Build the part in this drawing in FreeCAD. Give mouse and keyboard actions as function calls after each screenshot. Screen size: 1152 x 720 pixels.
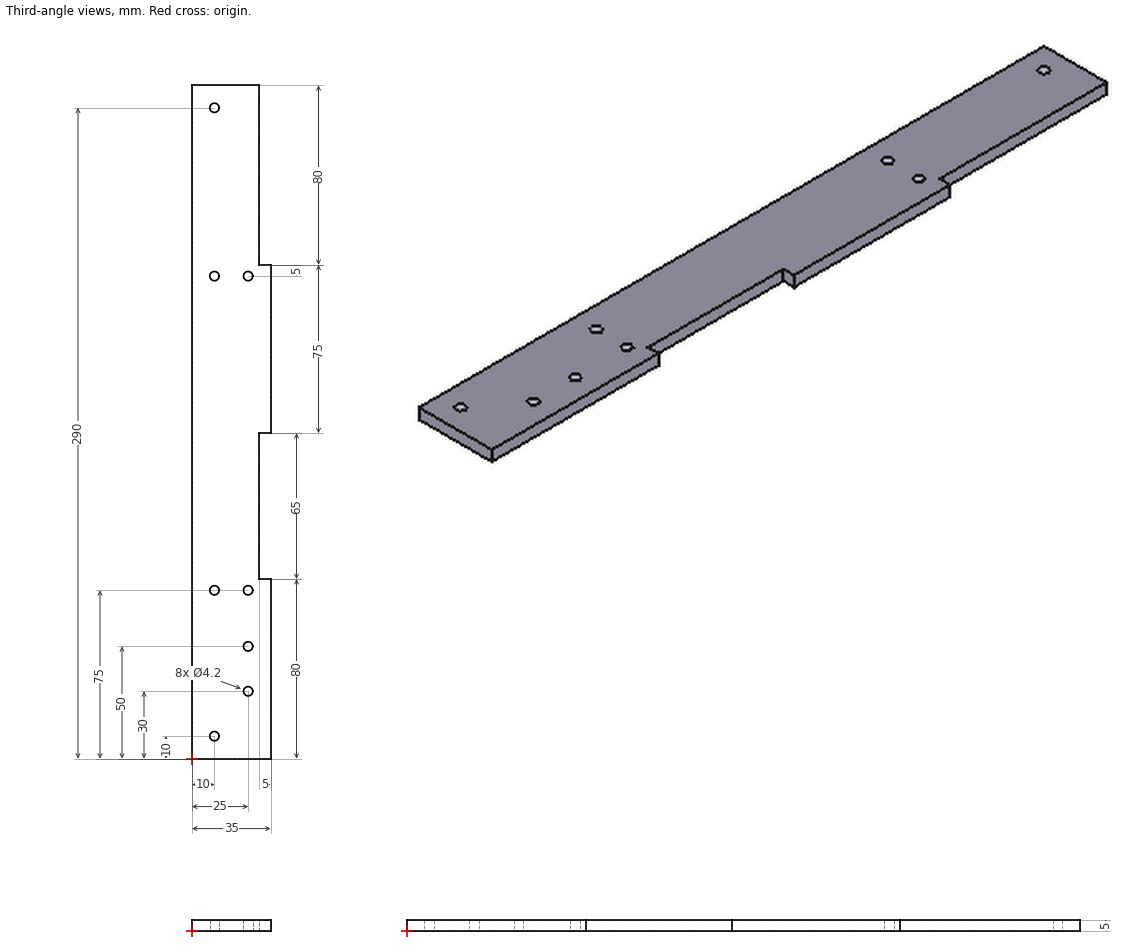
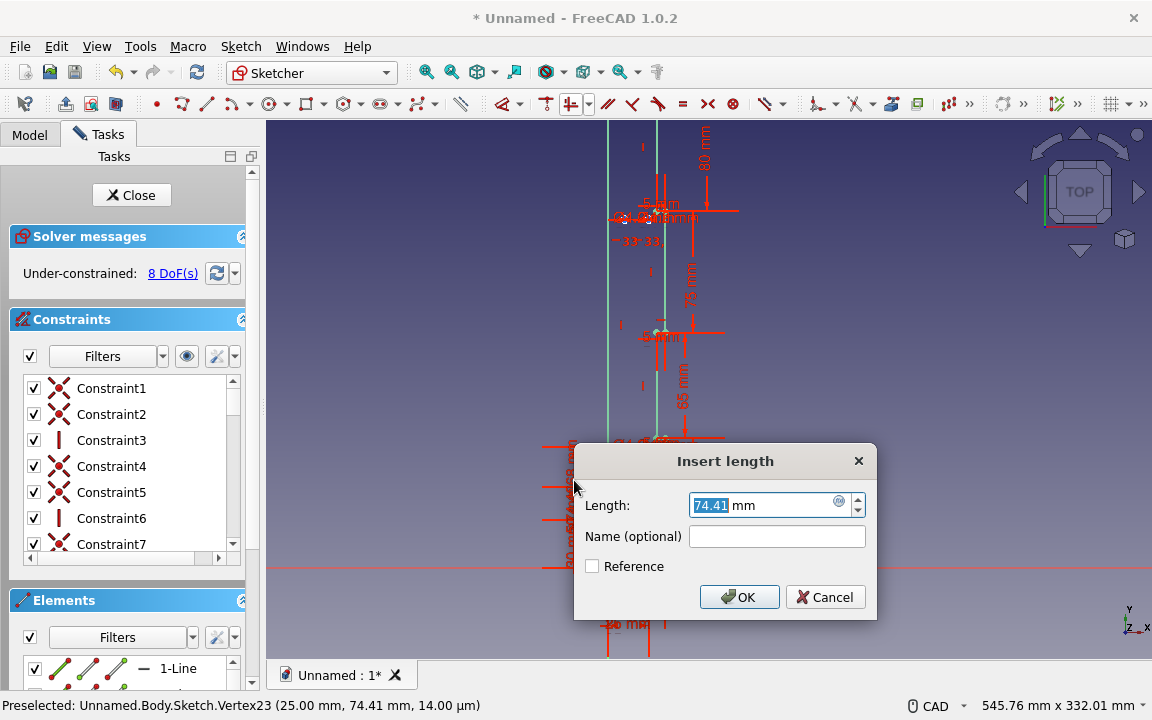
text(75)
key(Return)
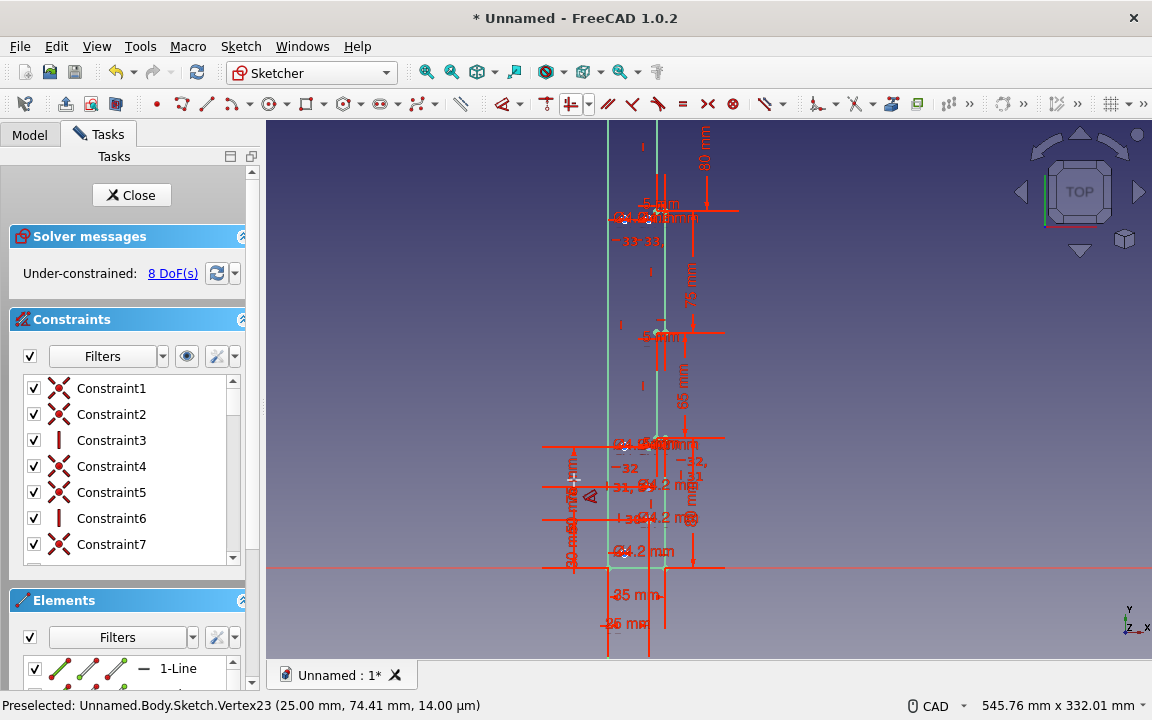
scroll(625, 553, up, 5)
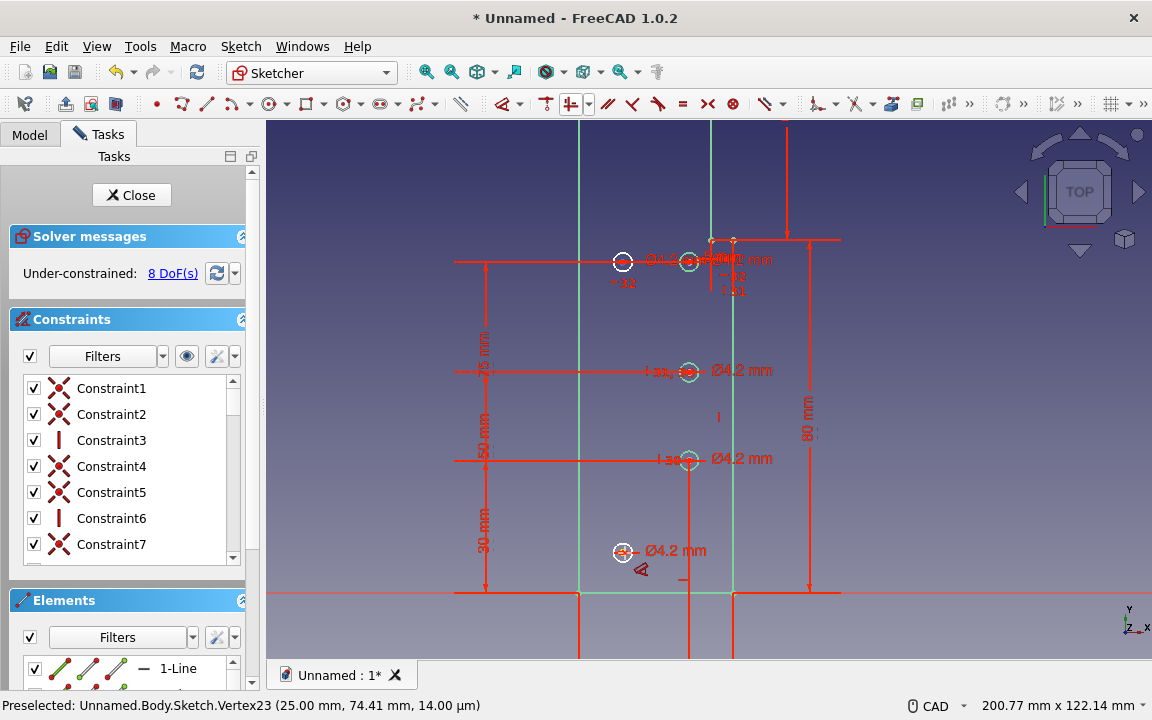
click(623, 553)
click(601, 627)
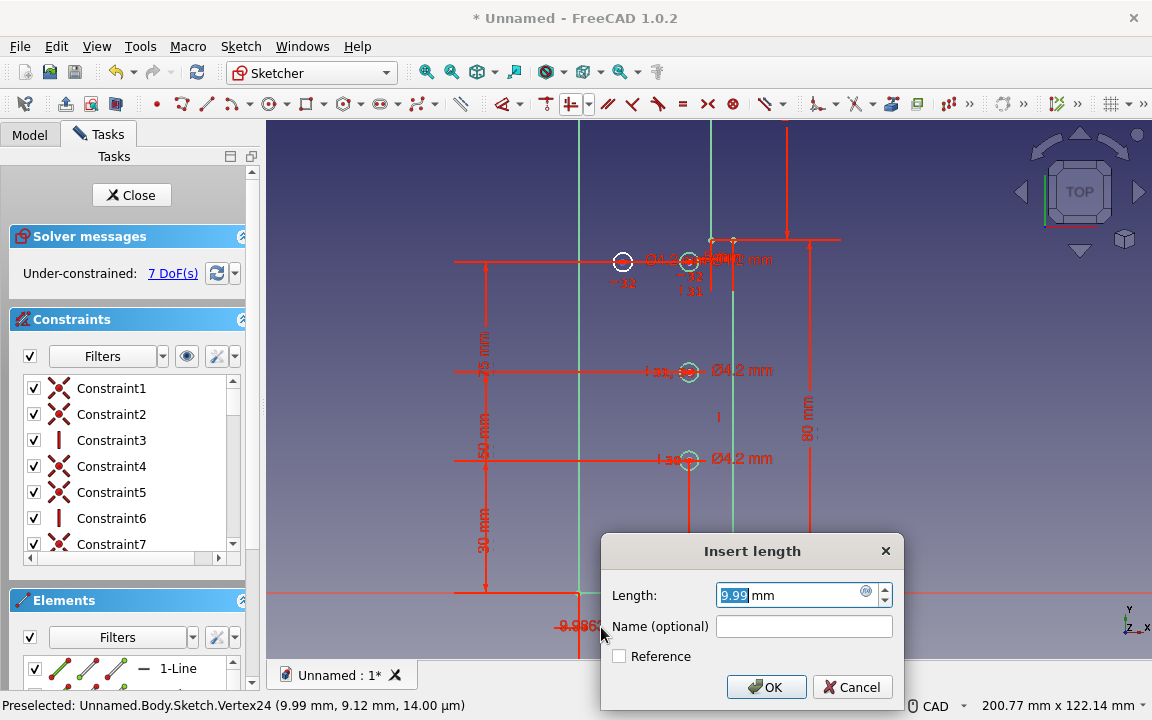
text(10)
key(Return)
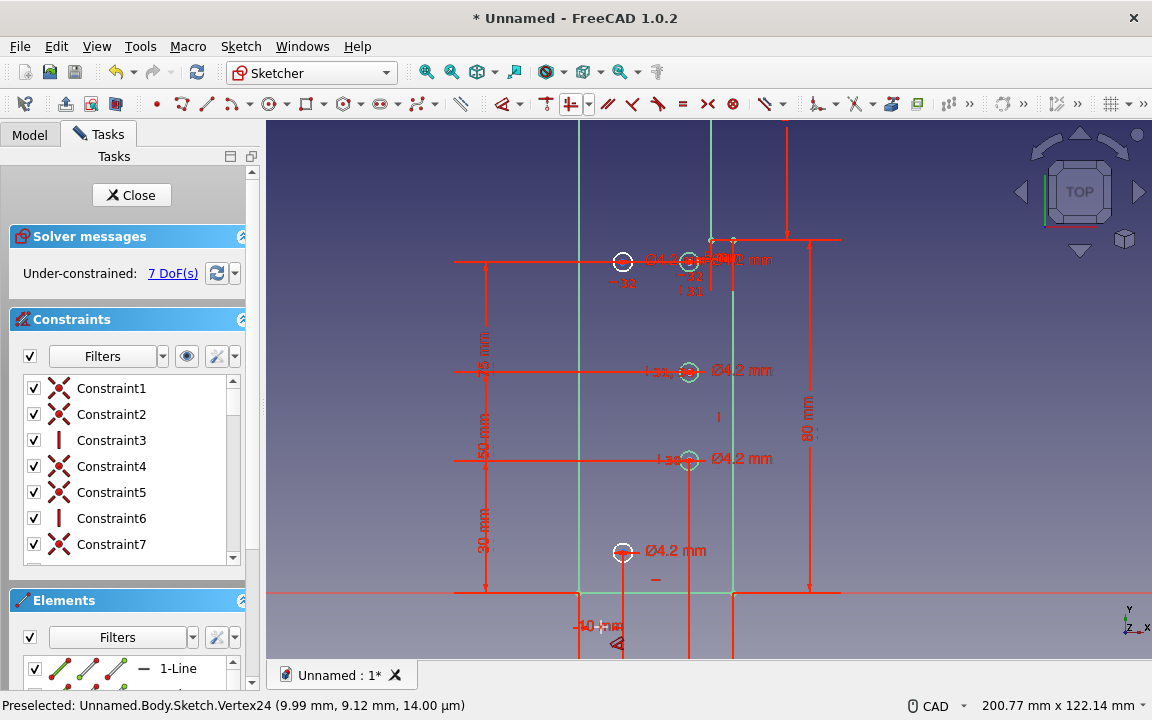
click(623, 553)
click(545, 573)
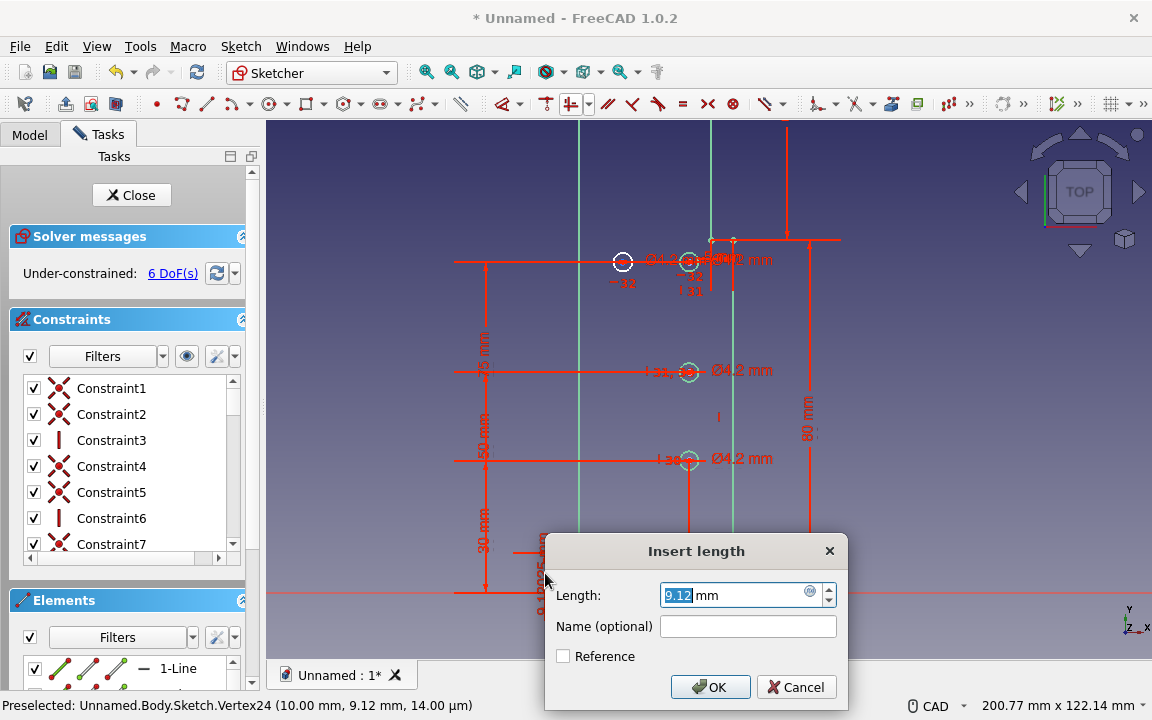
text(10)
key(Return)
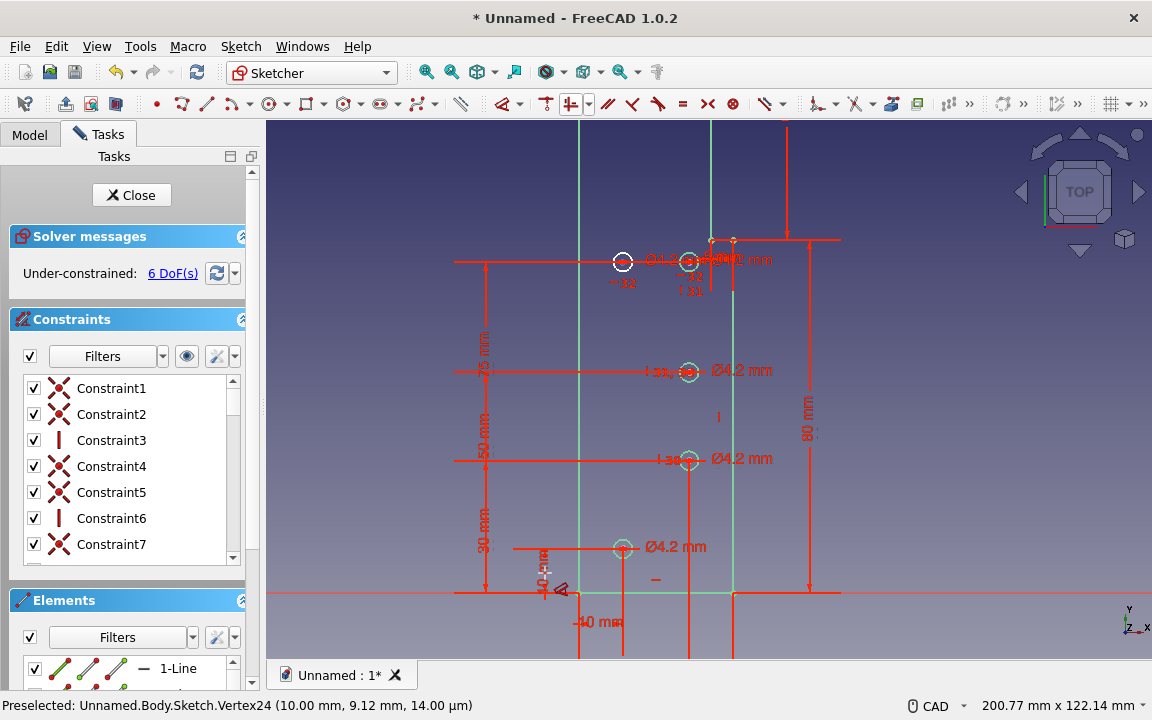
click(623, 262)
click(601, 228)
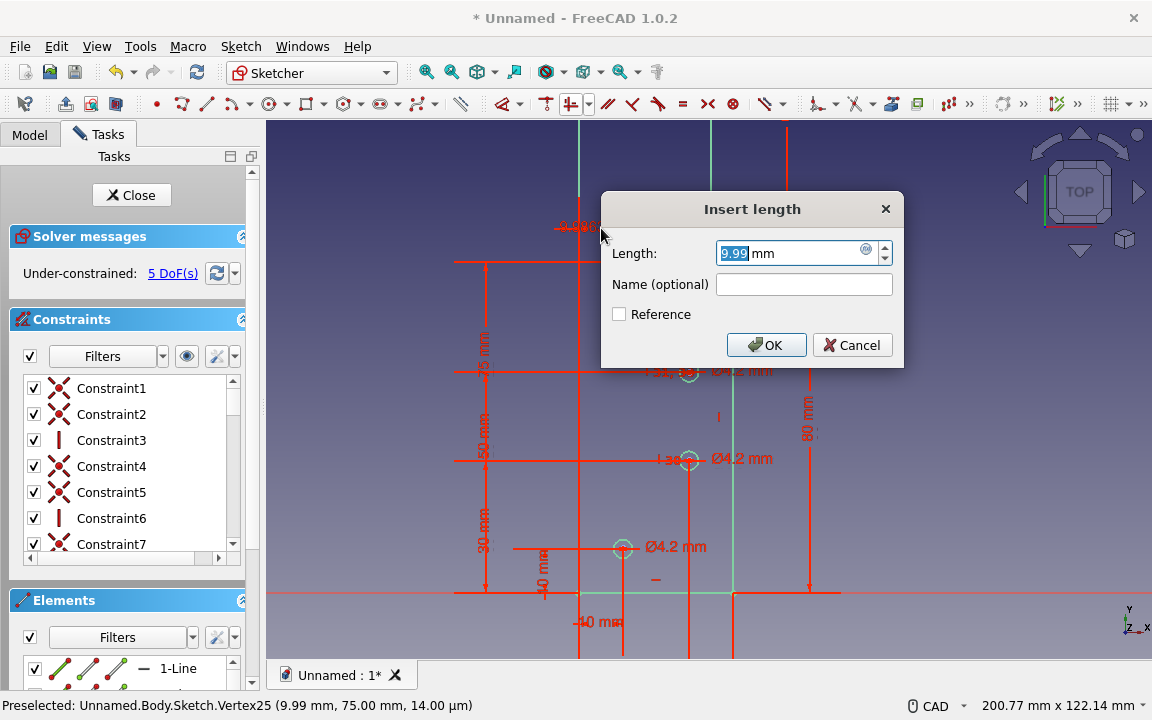
text(10)
key(Return)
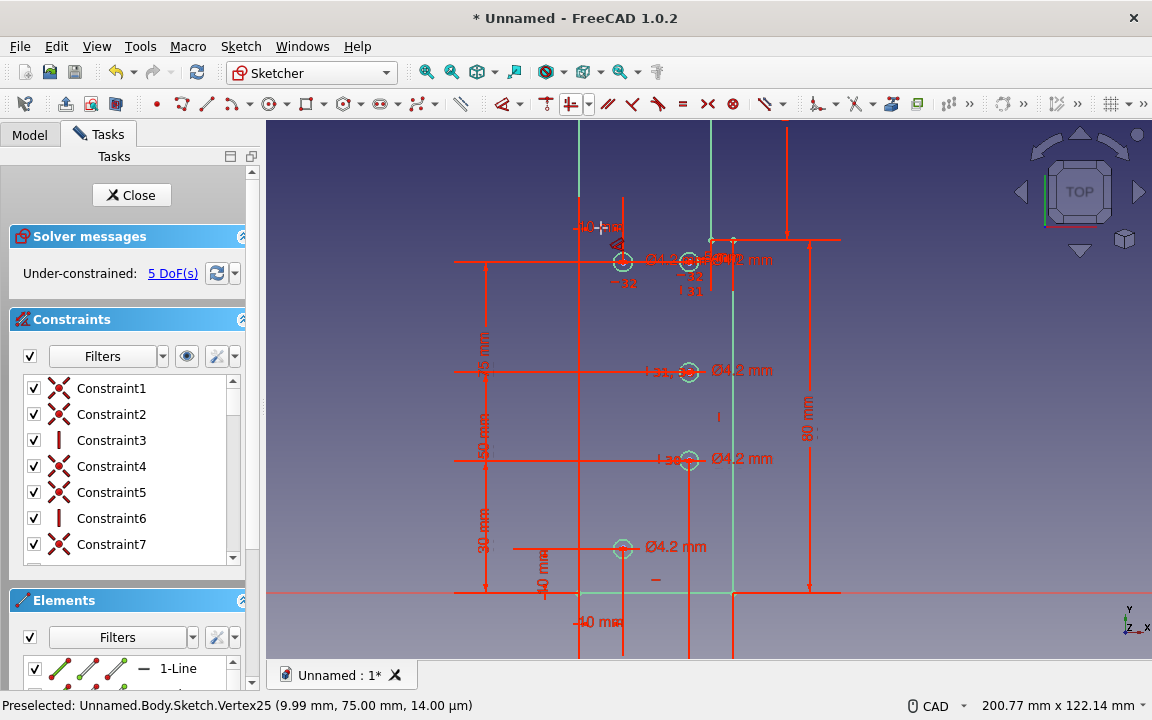
scroll(635, 540, down, 7)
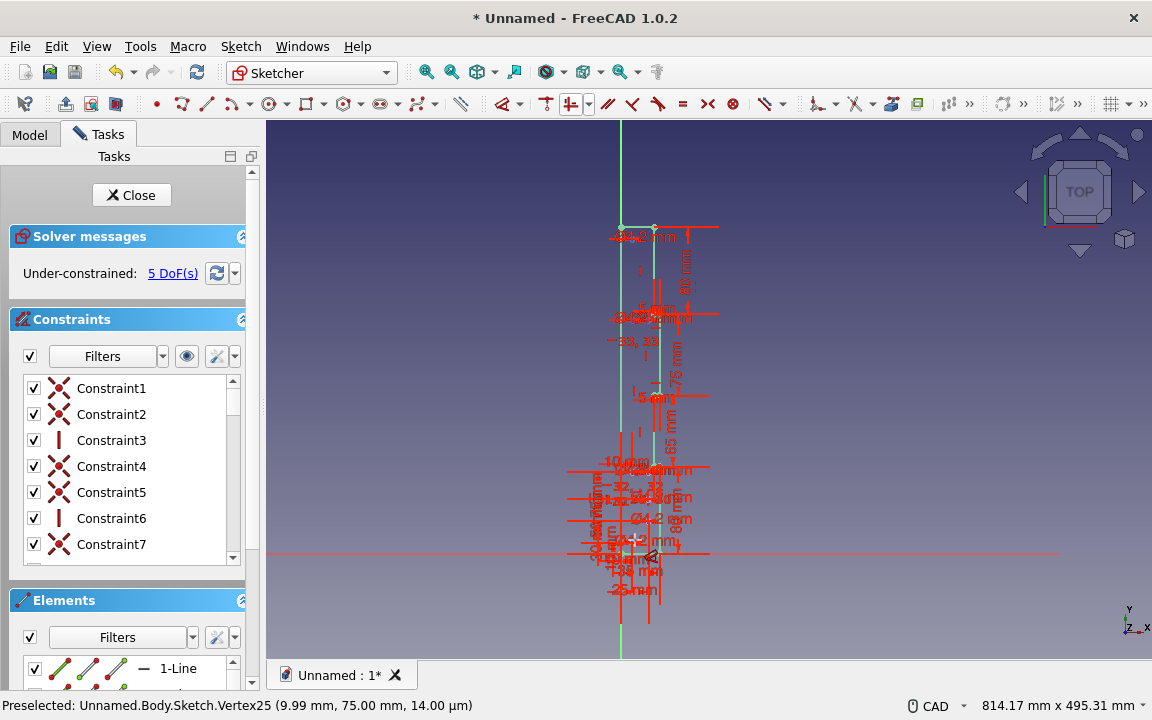
scroll(649, 320, up, 3)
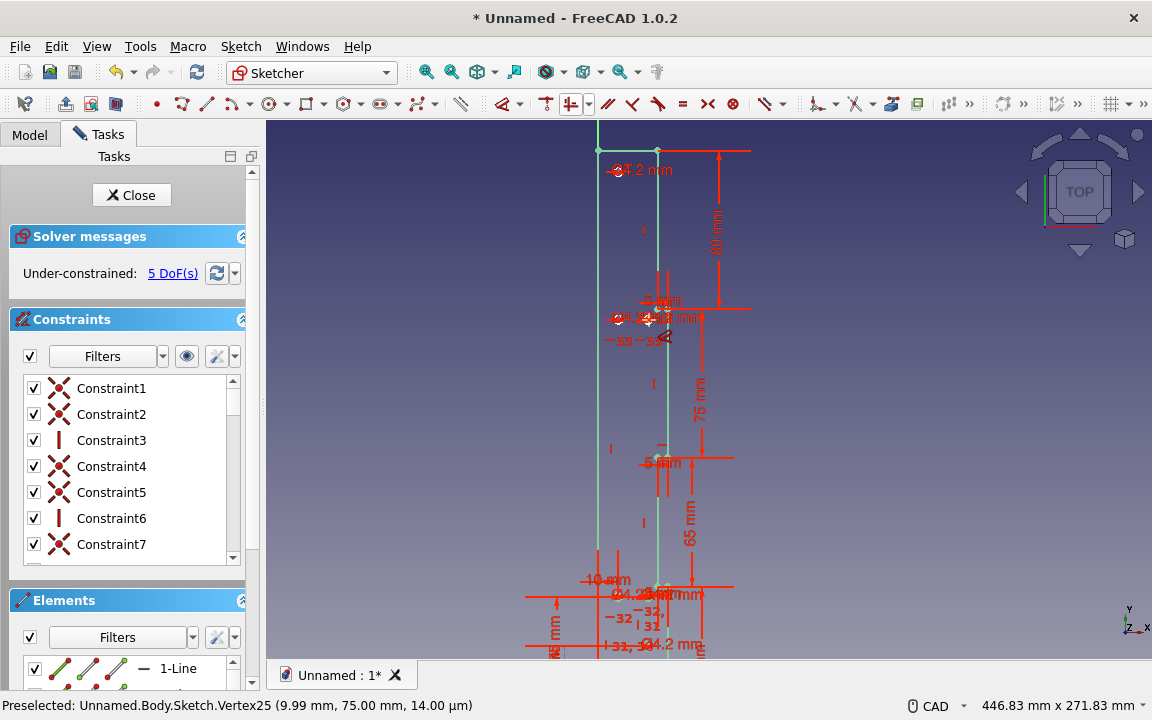
click(648, 320)
click(623, 262)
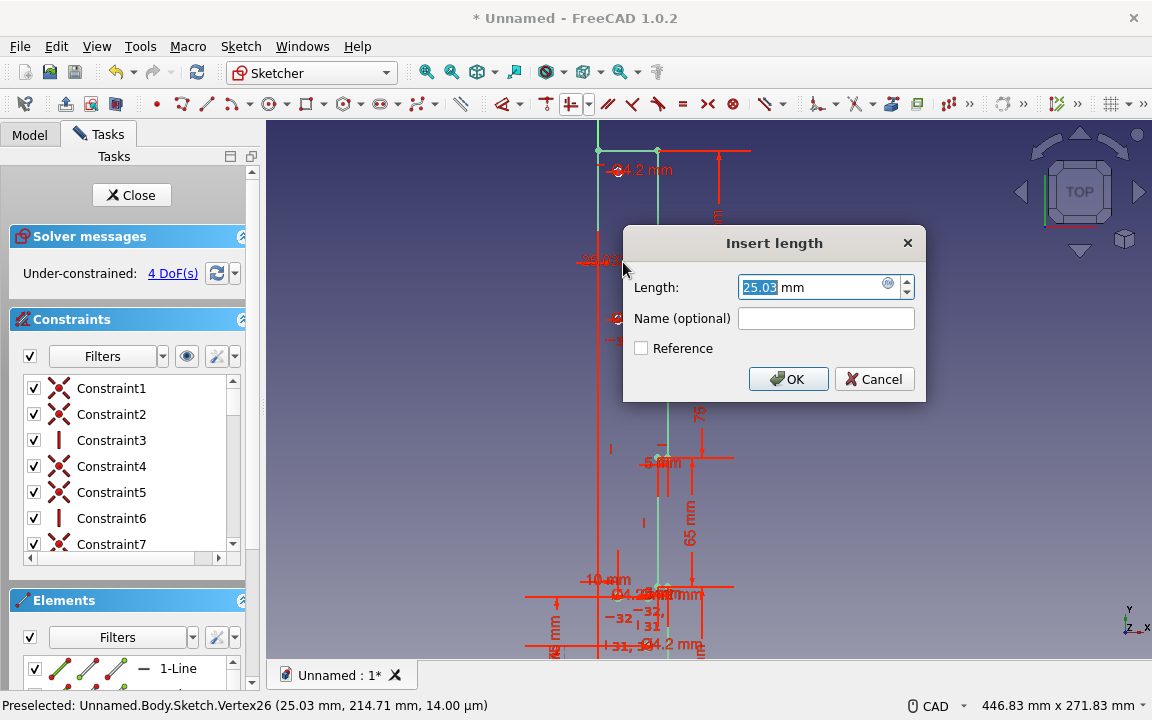
text(25)
key(Return)